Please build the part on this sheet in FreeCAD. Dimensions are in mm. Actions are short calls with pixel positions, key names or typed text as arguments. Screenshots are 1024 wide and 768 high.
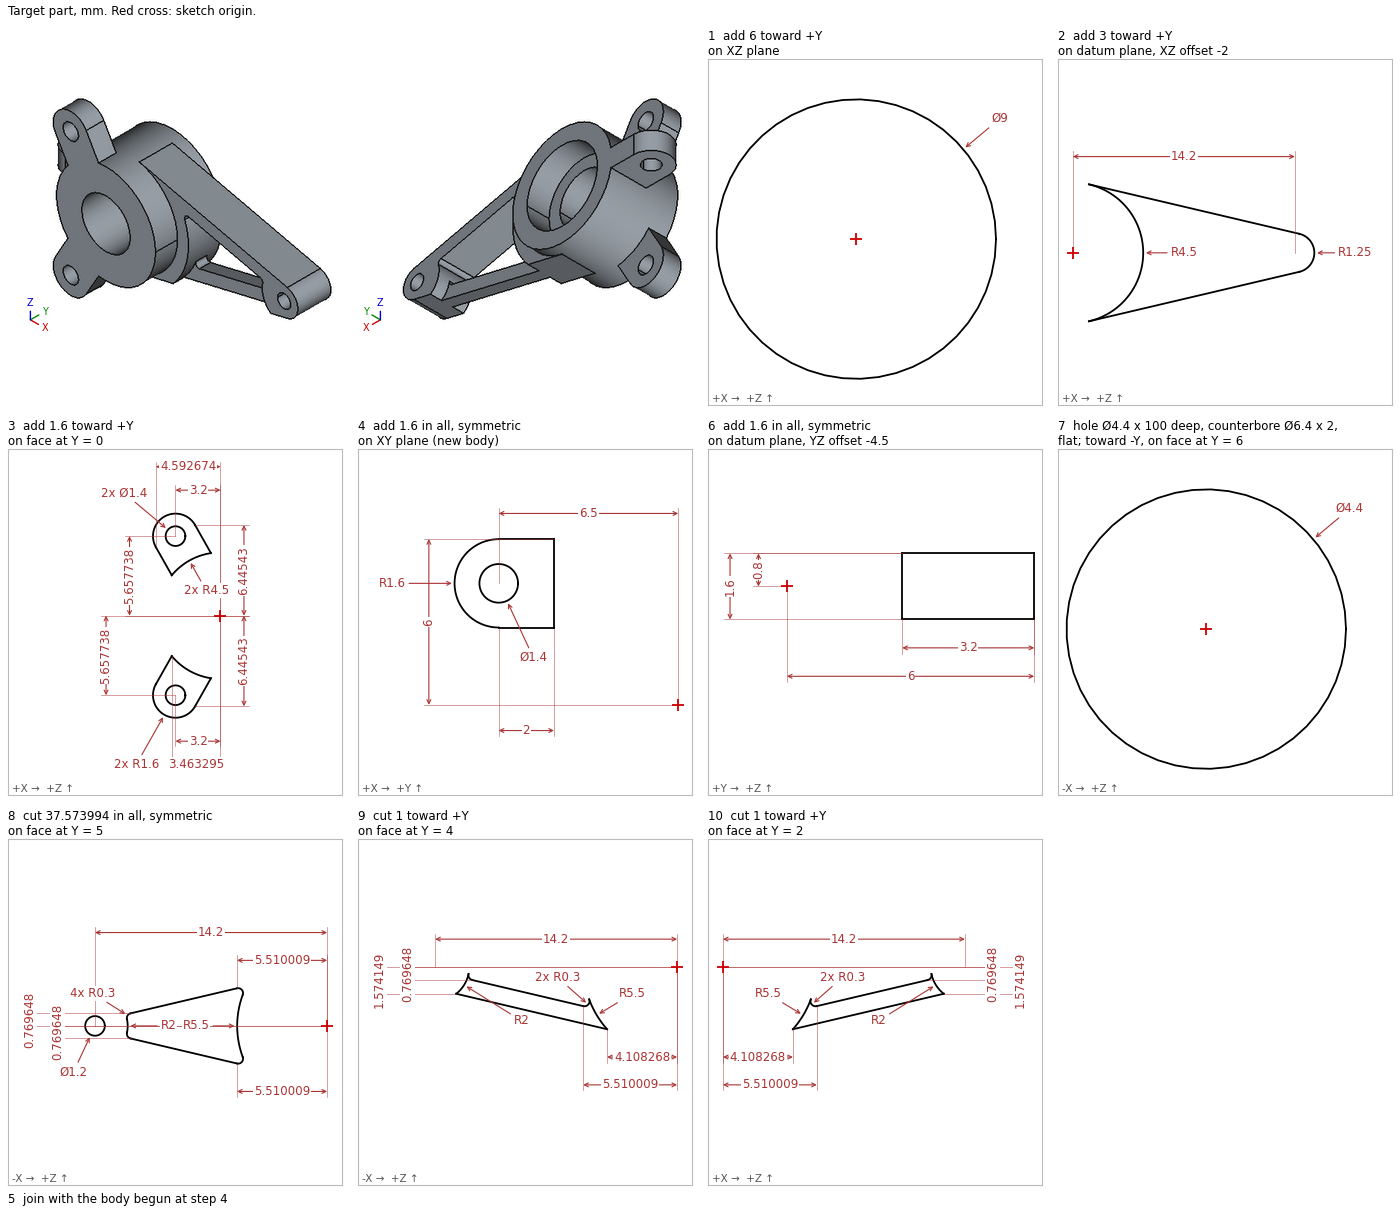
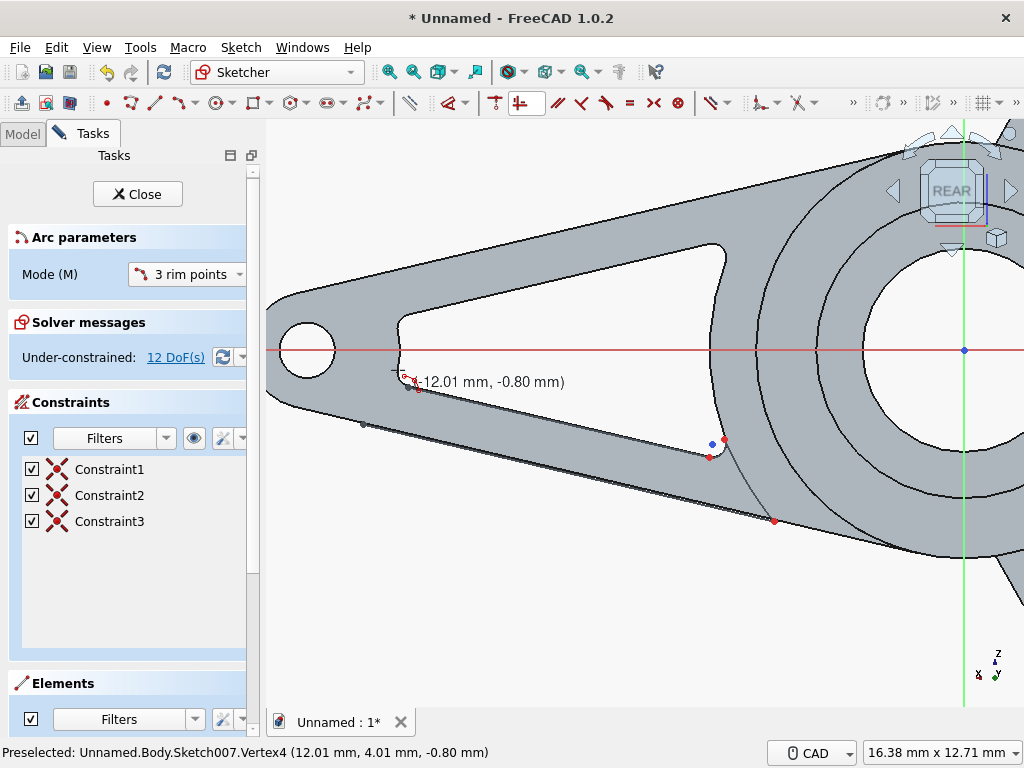
click(398, 370)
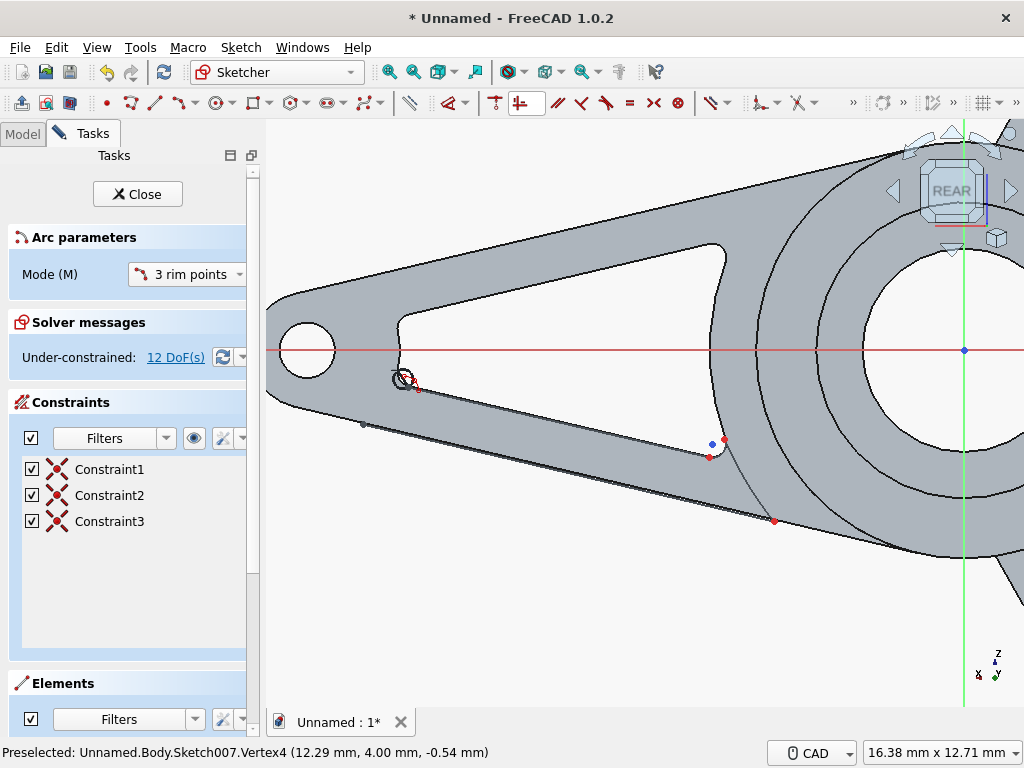
scroll(400, 380, up, 7)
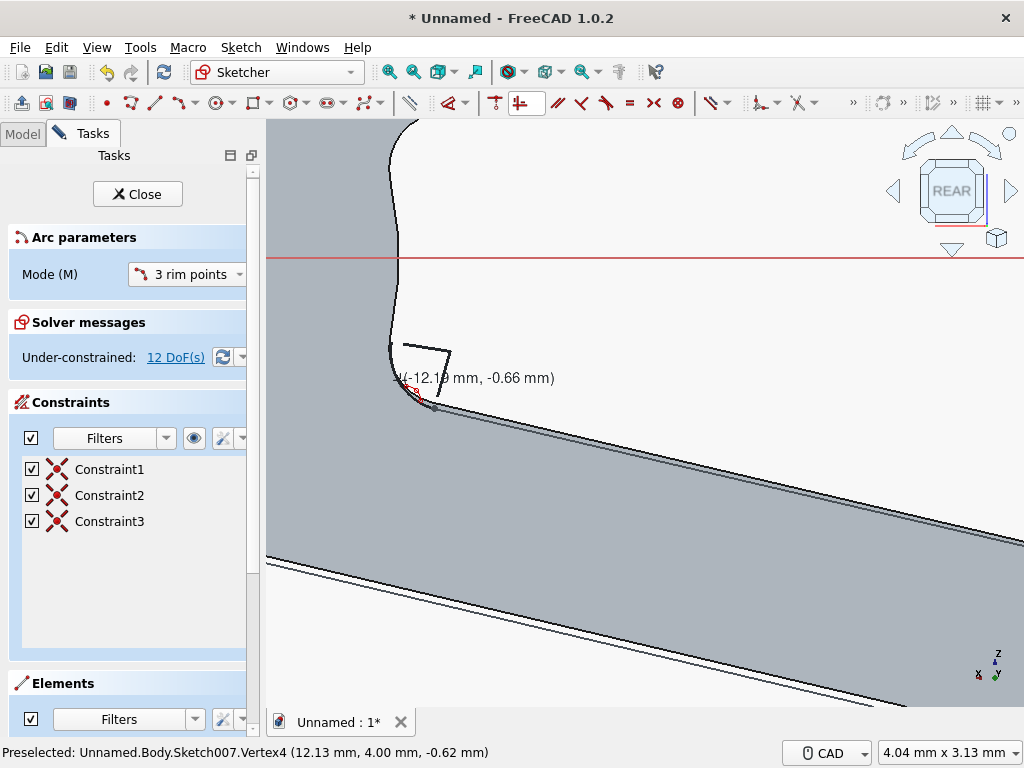
click(398, 378)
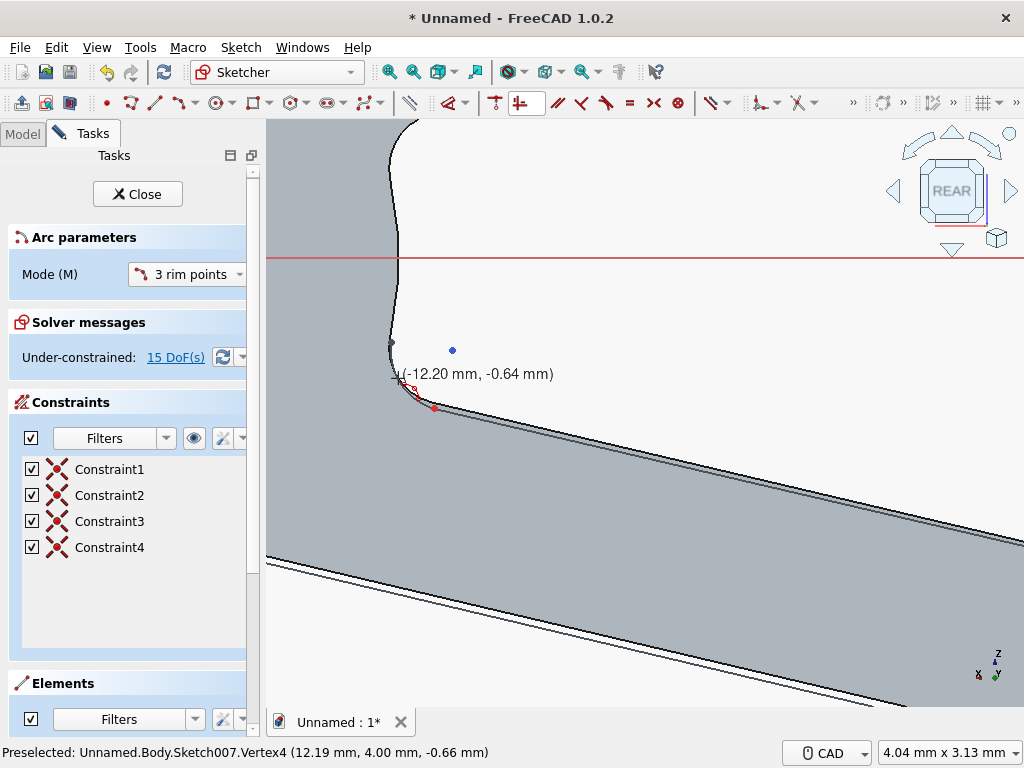
scroll(399, 376, down, 9)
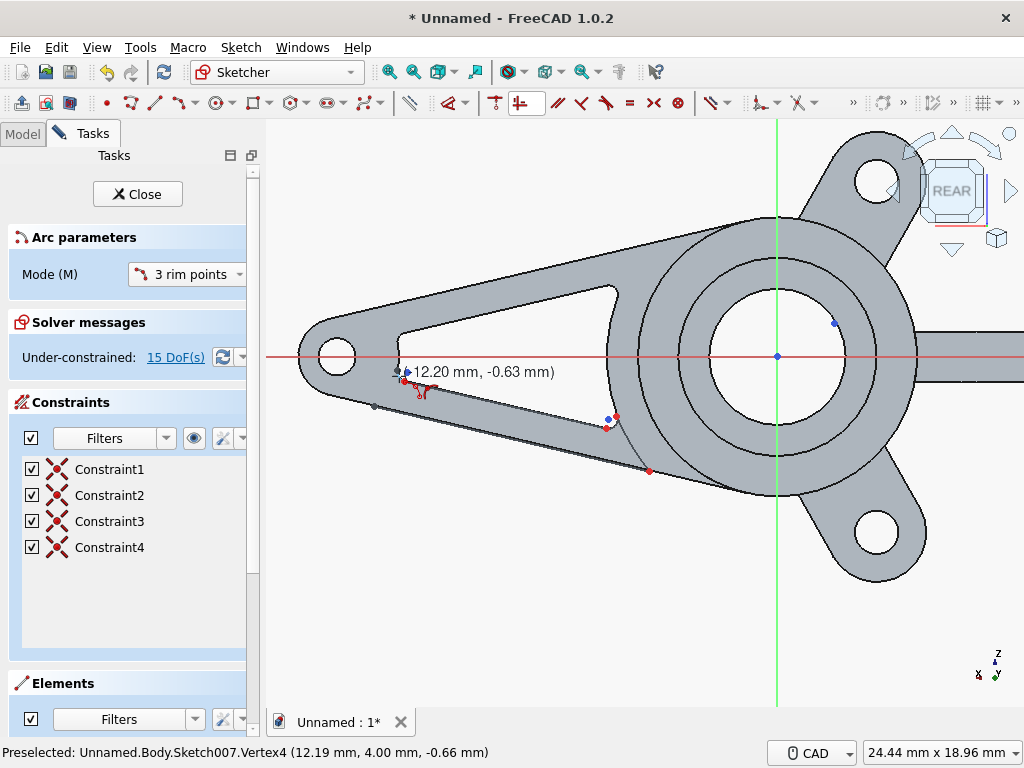
scroll(398, 370, up, 3)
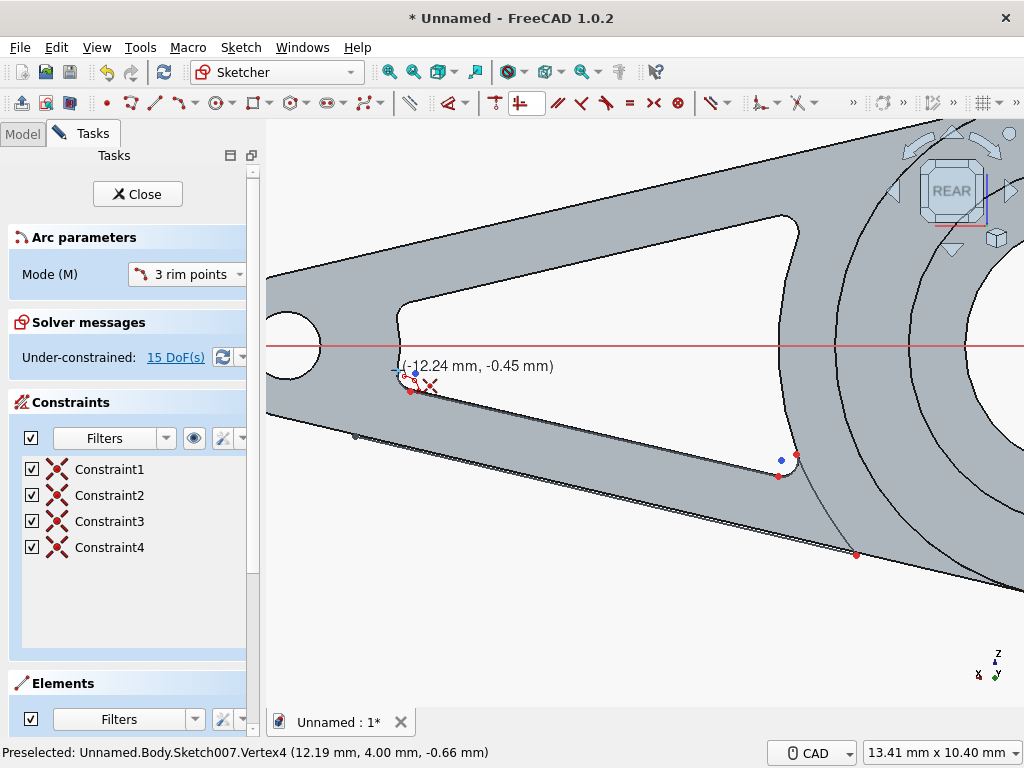
click(398, 371)
click(356, 437)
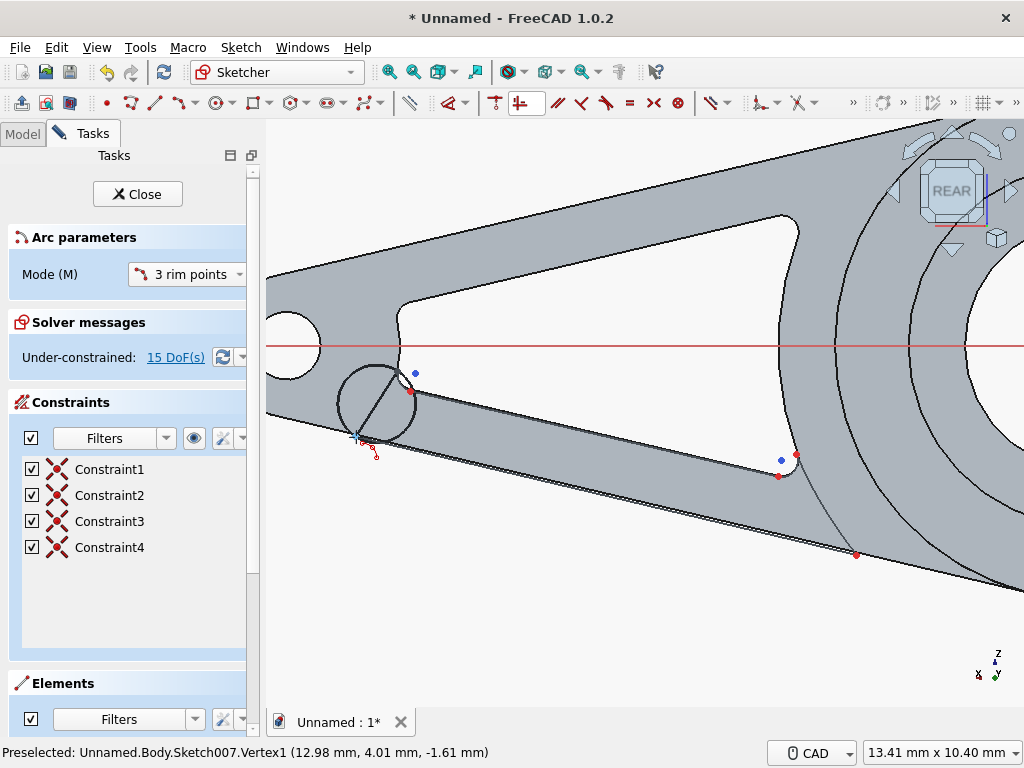
scroll(383, 406, up, 5)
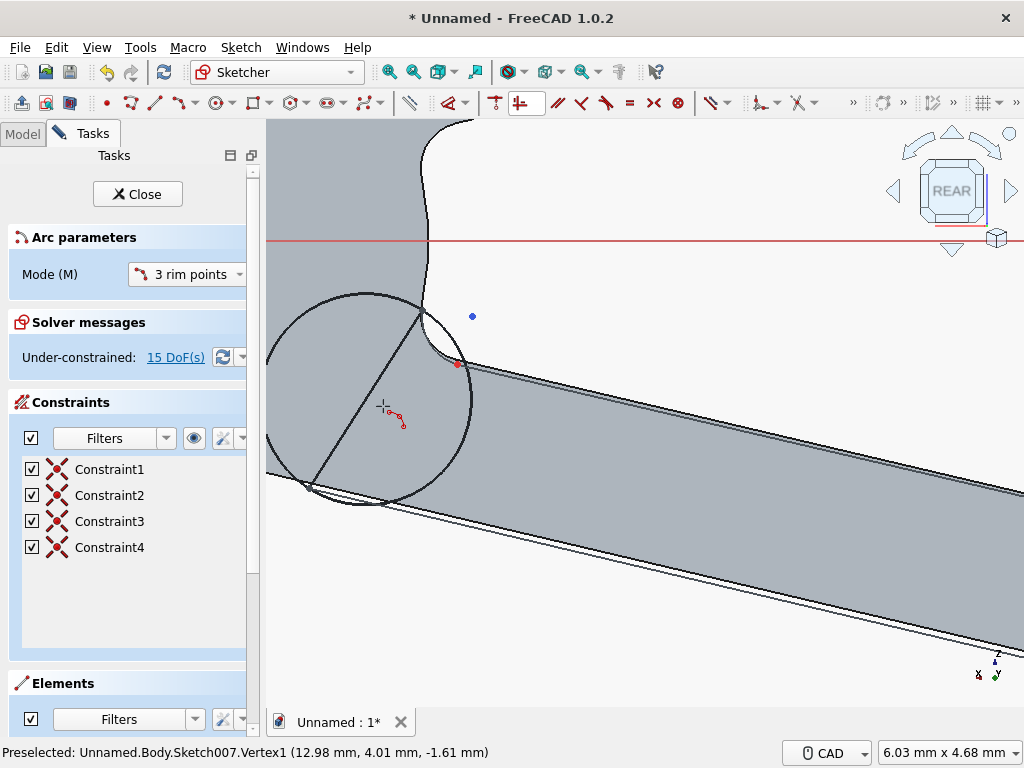
click(382, 404)
key(Escape)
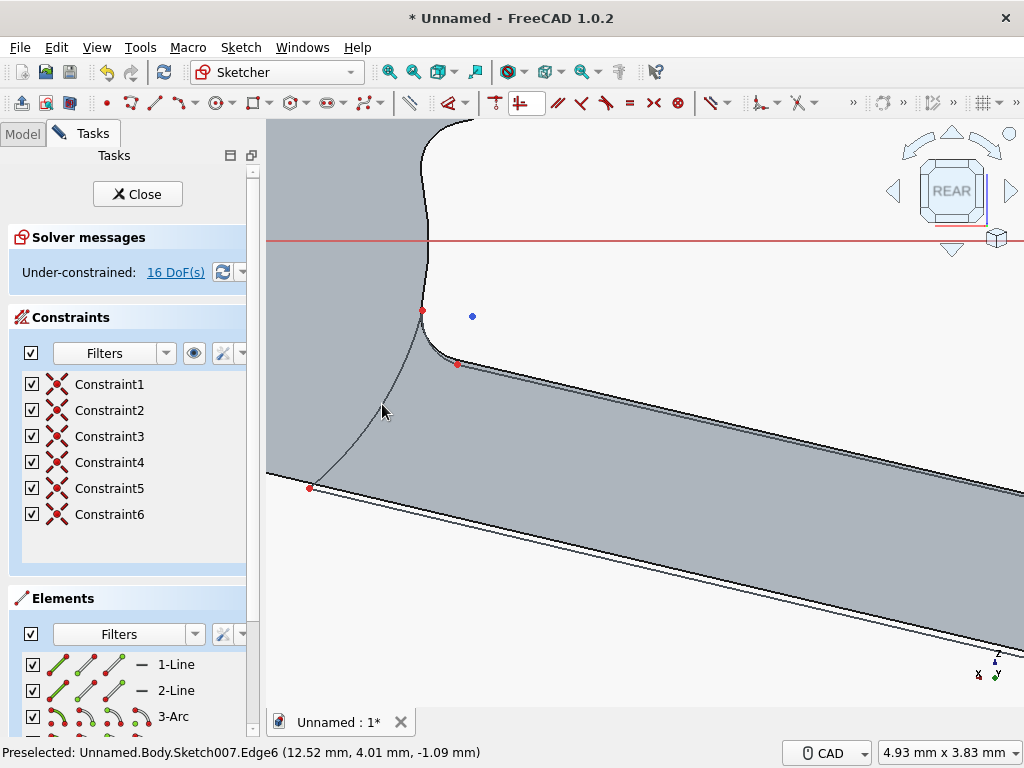
scroll(392, 385, down, 8)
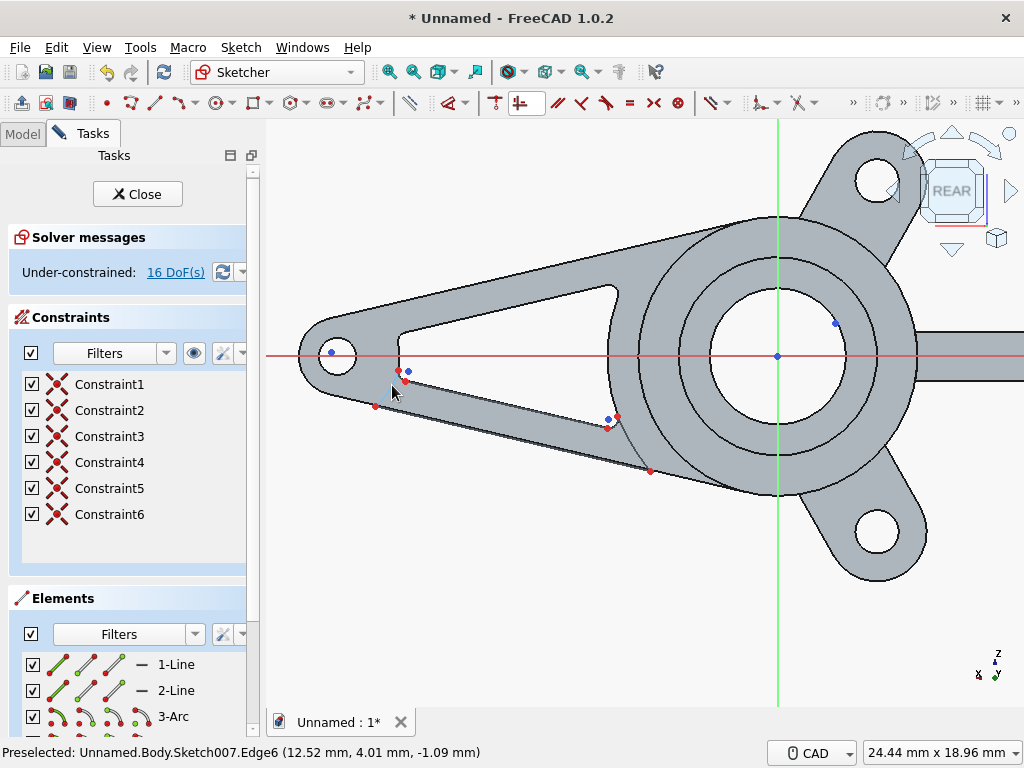
click(466, 395)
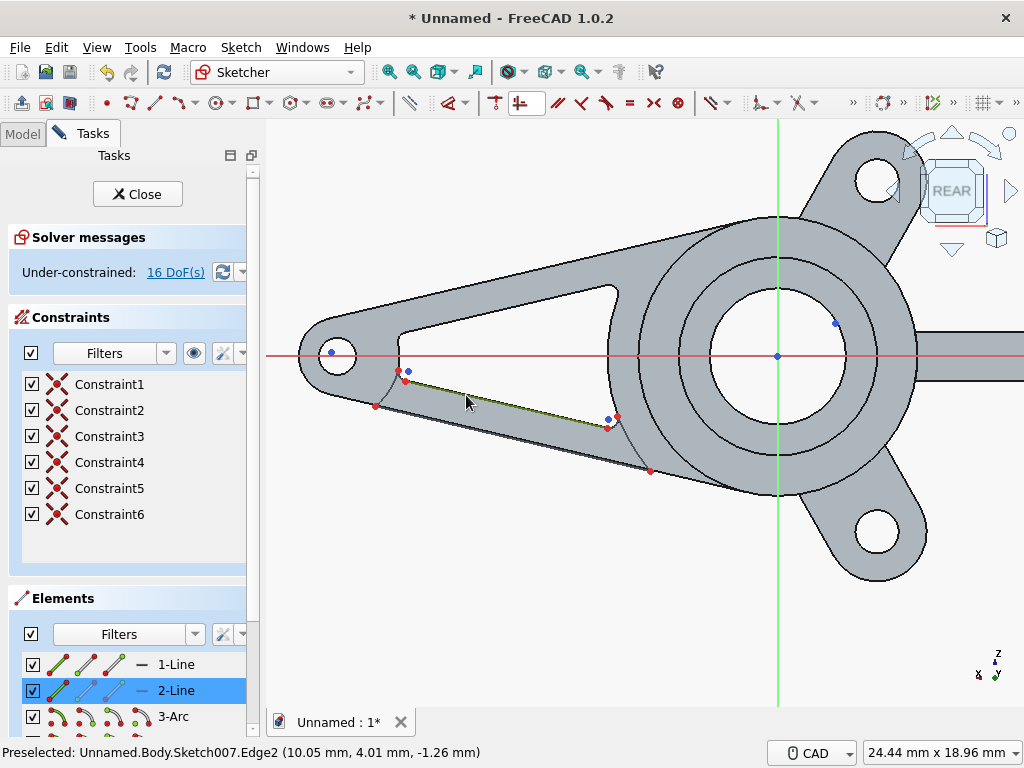
scroll(613, 428, up, 5)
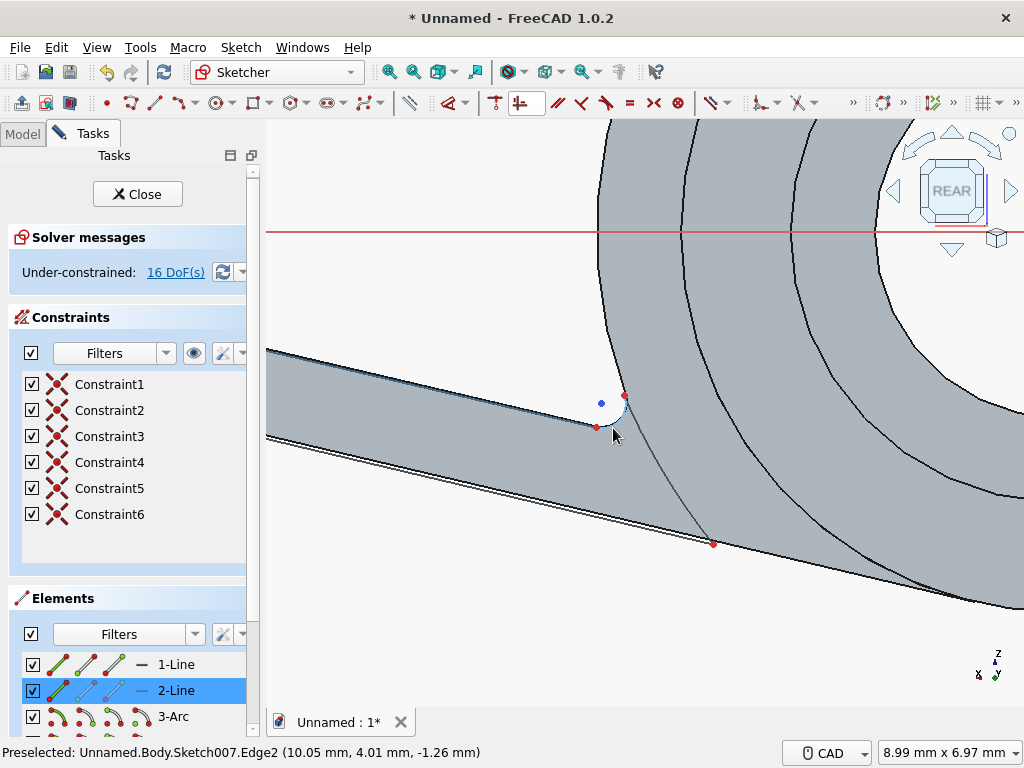
click(612, 426)